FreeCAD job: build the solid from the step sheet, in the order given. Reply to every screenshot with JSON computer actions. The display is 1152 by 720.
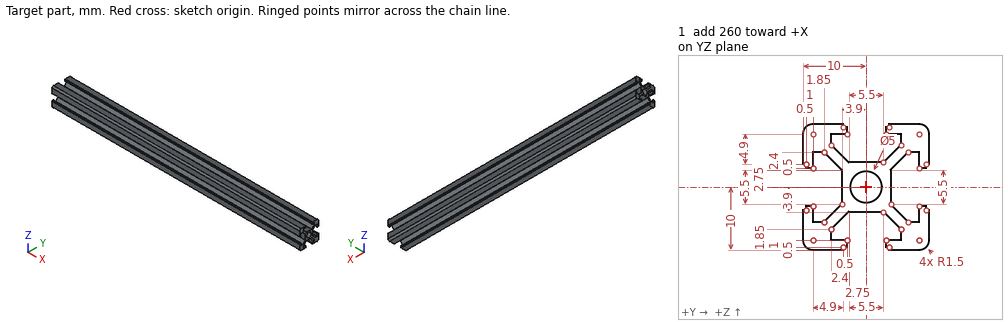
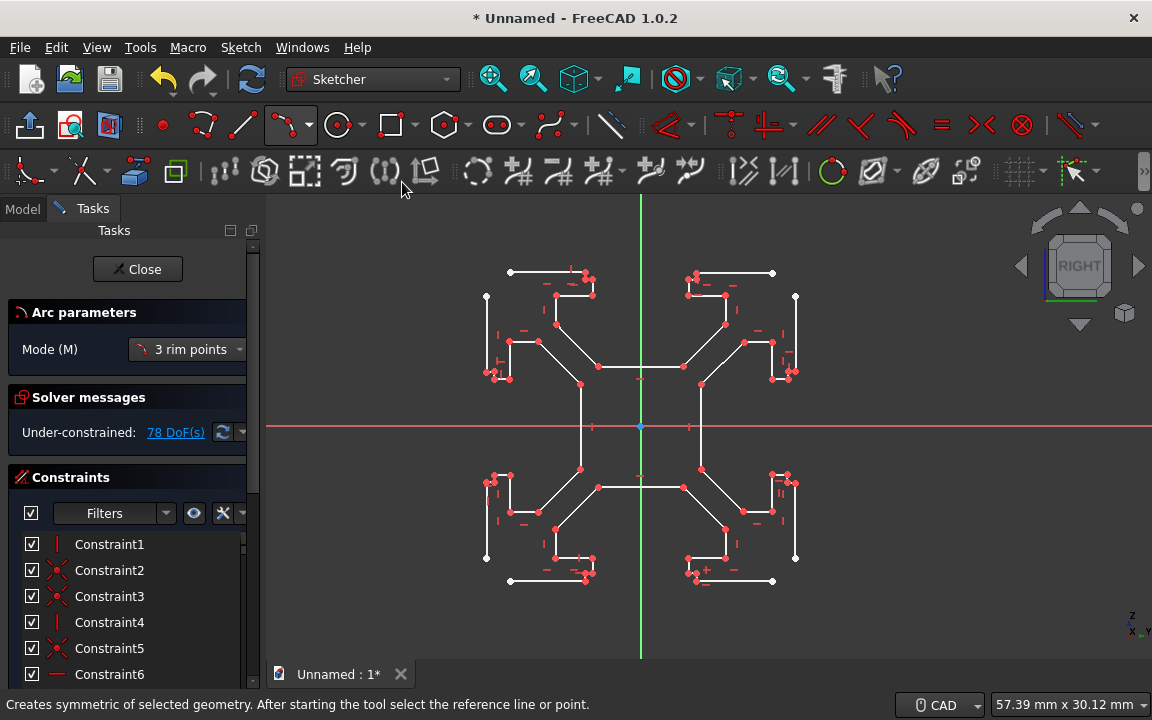
{"action": "left_click", "coordinate": [487, 558]}
{"action": "left_click", "coordinate": [510, 581]}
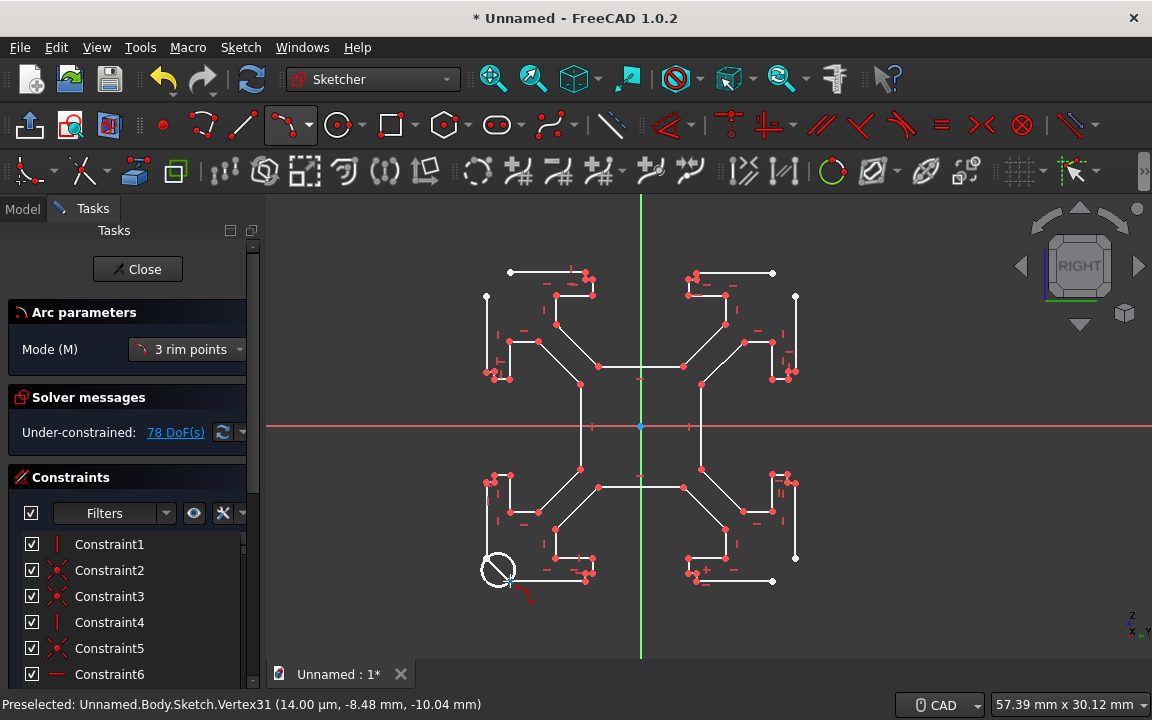
{"action": "scroll", "coordinate": [493, 574], "scroll_direction": "up", "scroll_amount": 5}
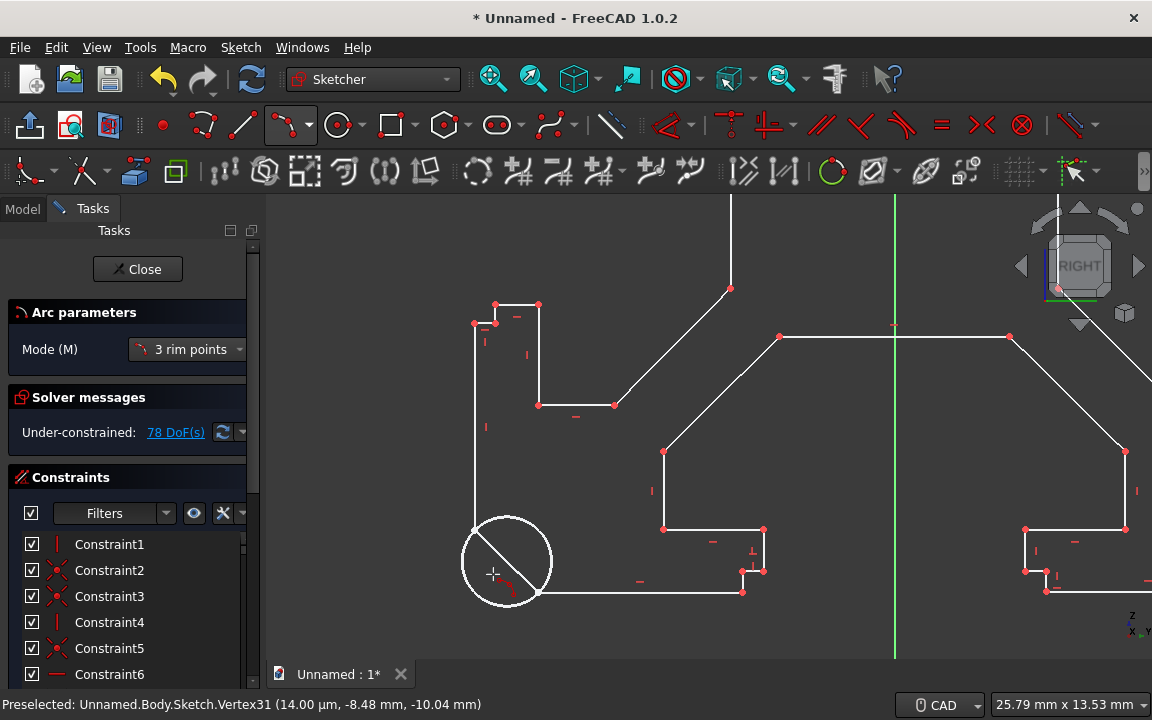
{"action": "left_click", "coordinate": [493, 573]}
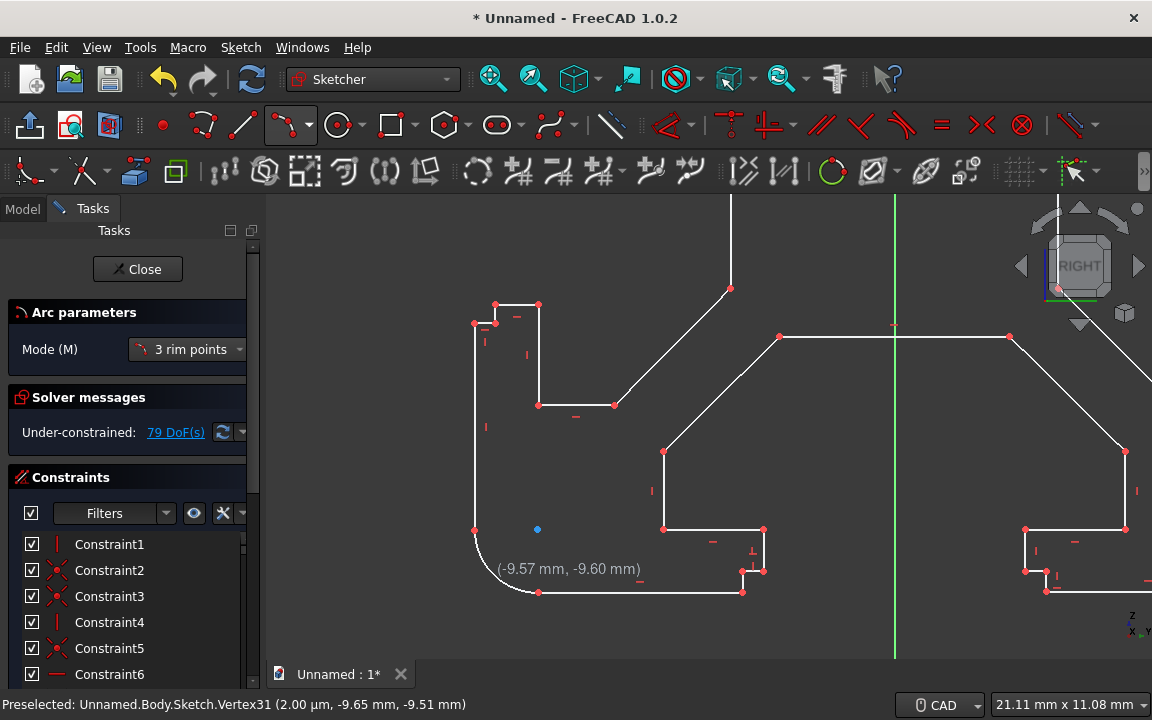
{"action": "scroll", "coordinate": [493, 575], "scroll_direction": "down", "scroll_amount": 5}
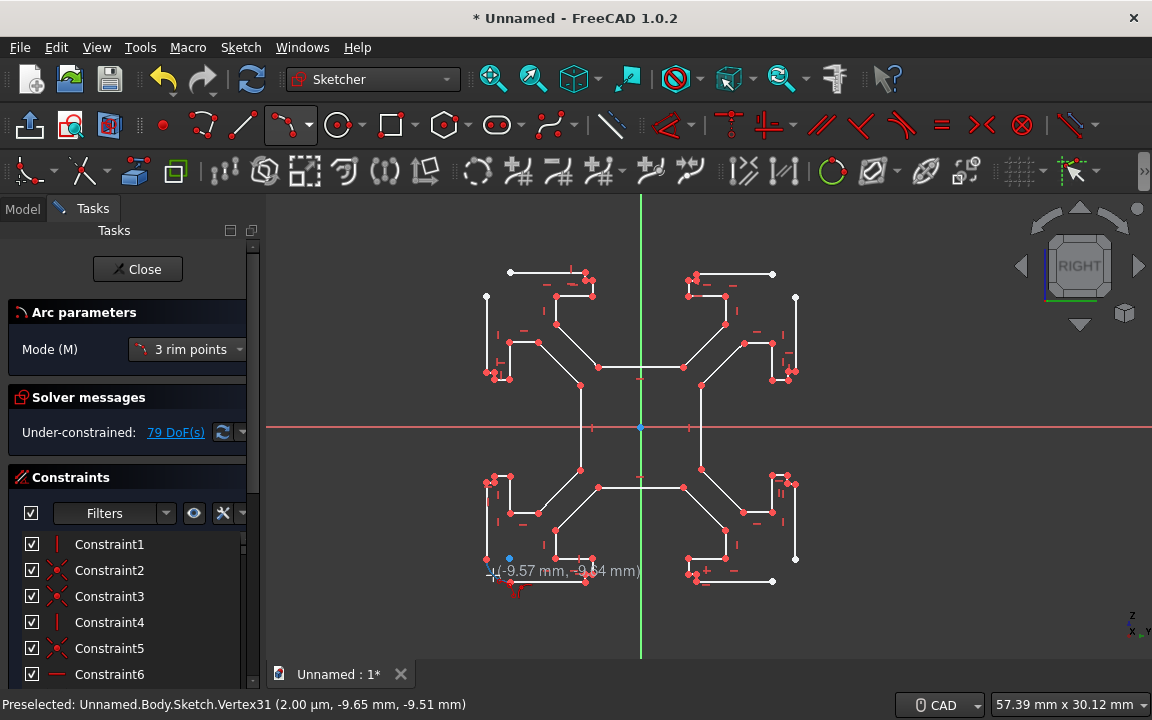
{"action": "left_click", "coordinate": [772, 582]}
{"action": "left_click", "coordinate": [795, 559]}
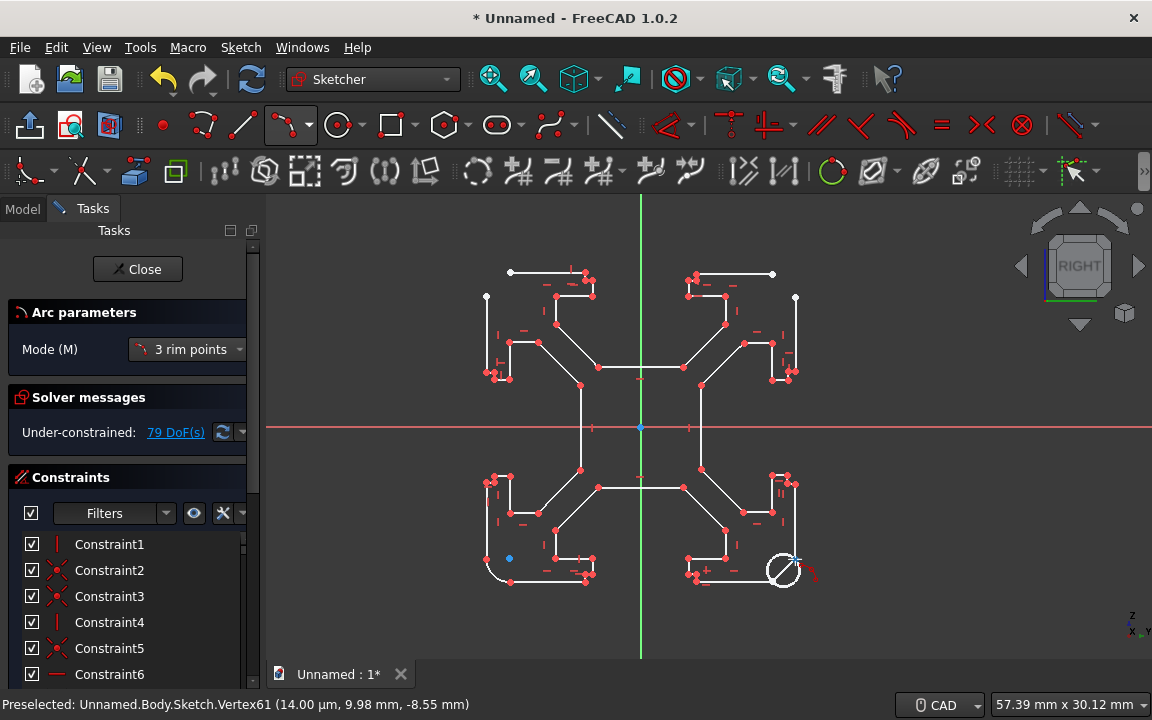
{"action": "scroll", "coordinate": [789, 575], "scroll_direction": "up", "scroll_amount": 5}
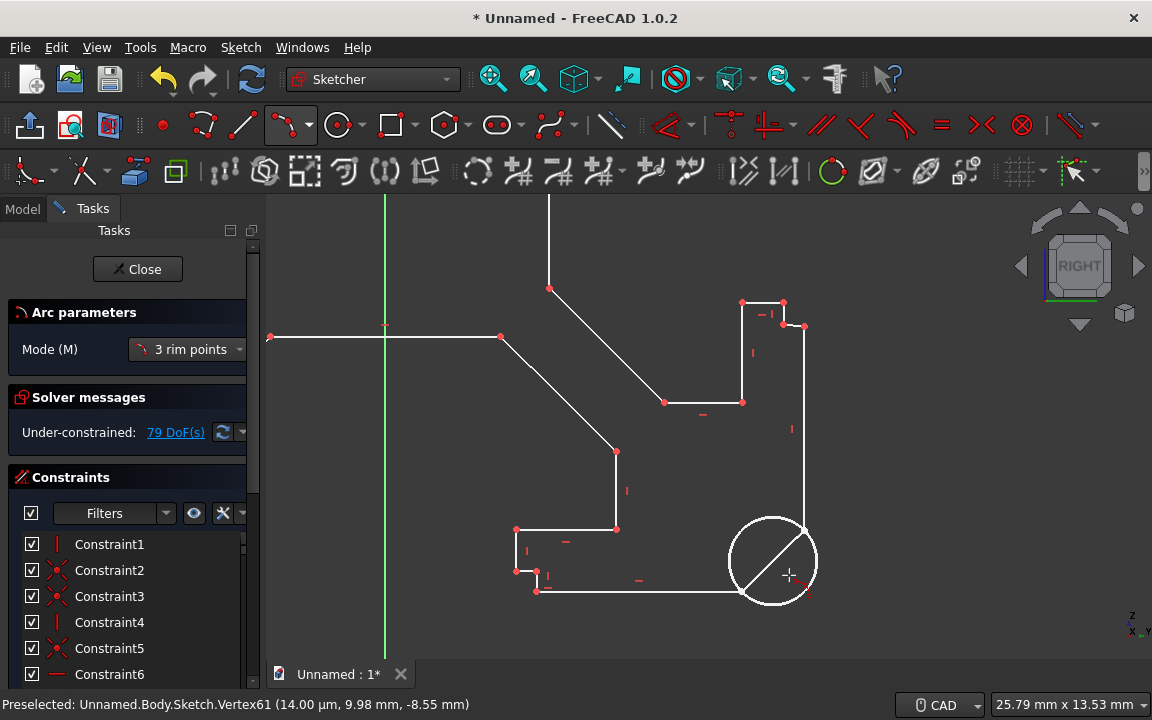
{"action": "left_click", "coordinate": [787, 573]}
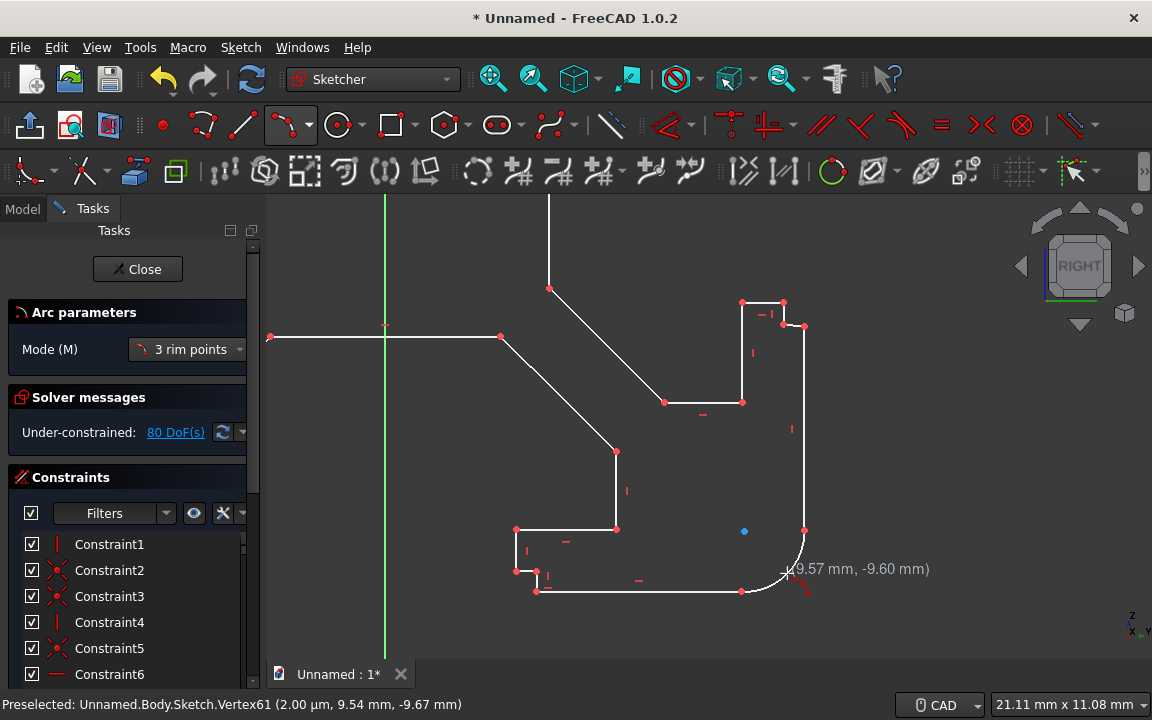
{"action": "scroll", "coordinate": [789, 575], "scroll_direction": "down", "scroll_amount": 5}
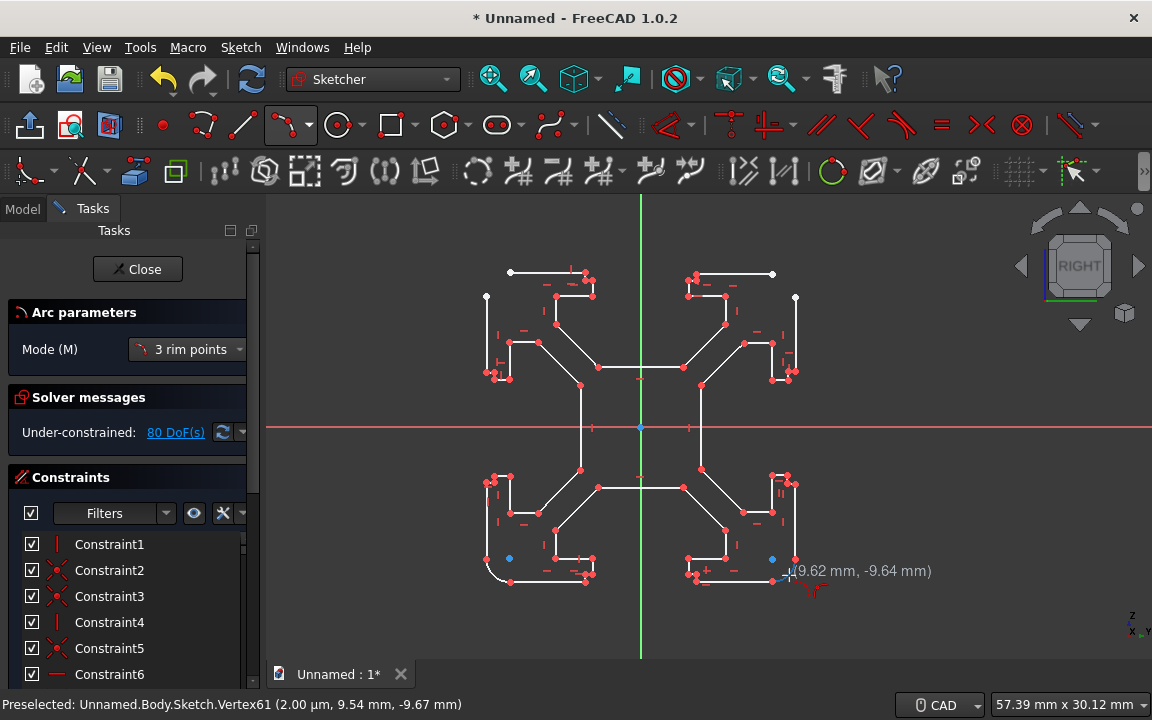
{"action": "left_click", "coordinate": [796, 297]}
{"action": "left_click", "coordinate": [772, 274]}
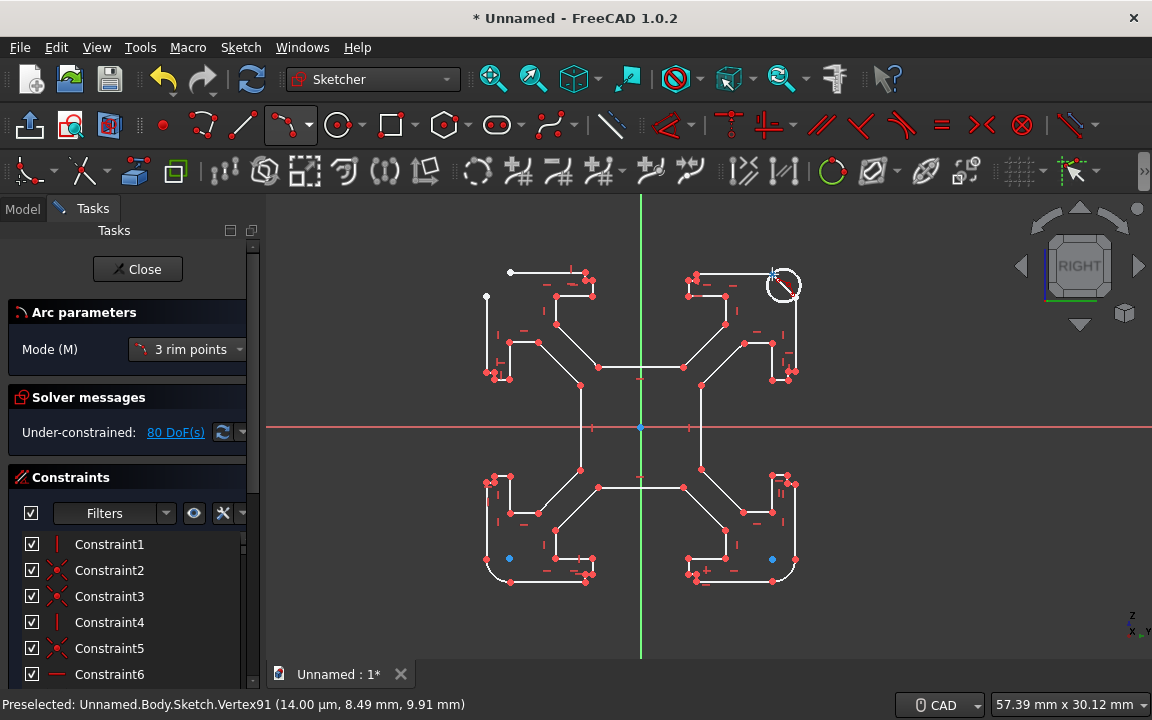
{"action": "scroll", "coordinate": [789, 279], "scroll_direction": "up", "scroll_amount": 5}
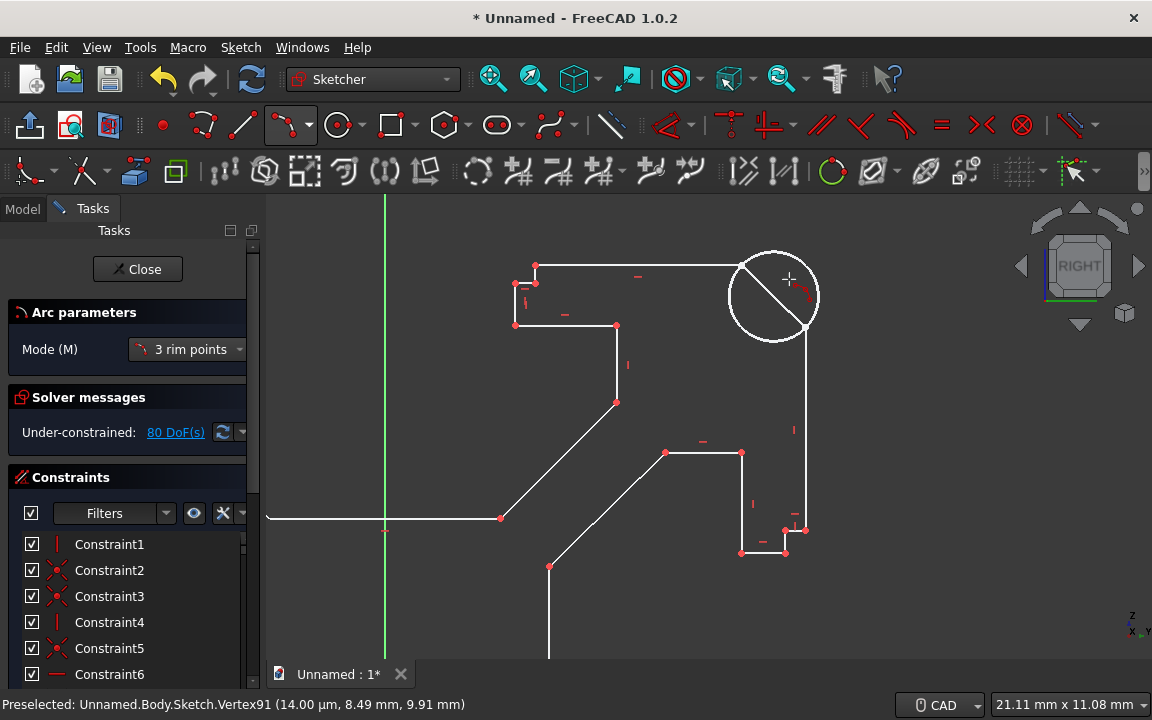
{"action": "left_click", "coordinate": [787, 280]}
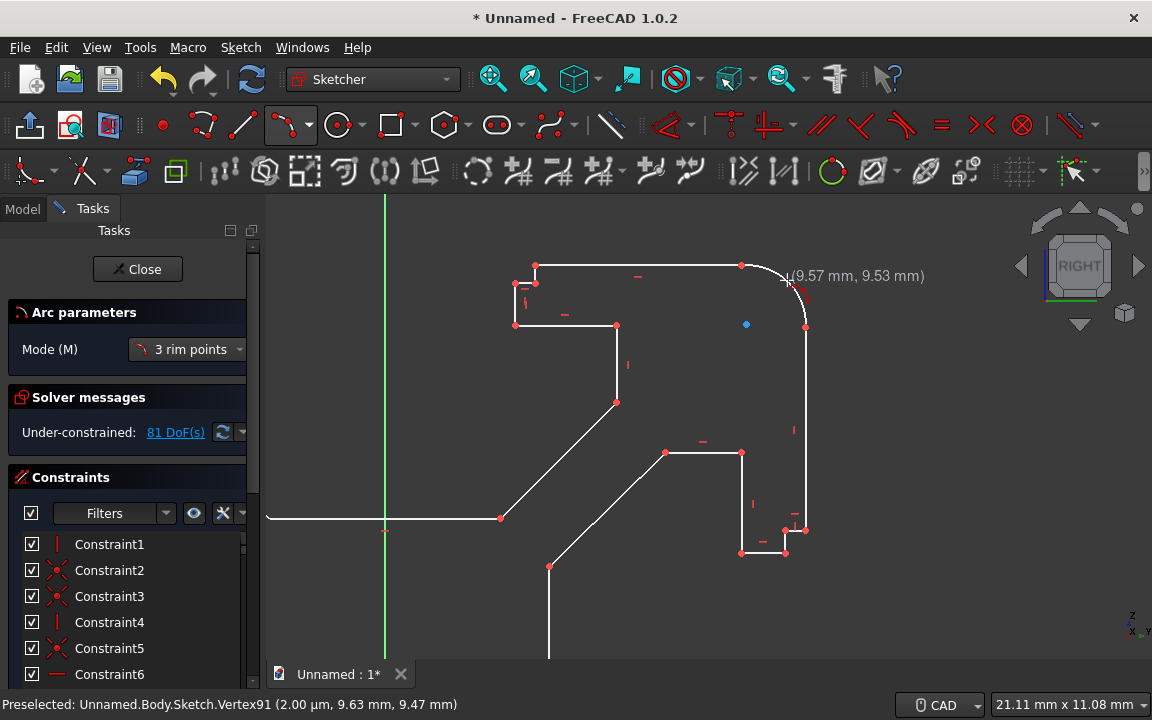
{"action": "scroll", "coordinate": [789, 278], "scroll_direction": "down", "scroll_amount": 5}